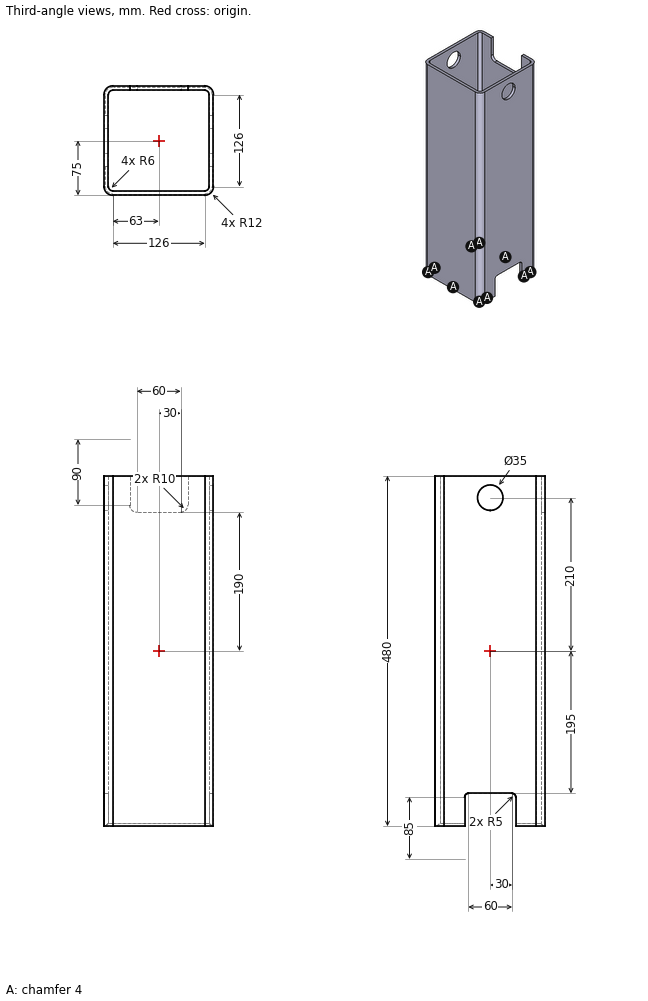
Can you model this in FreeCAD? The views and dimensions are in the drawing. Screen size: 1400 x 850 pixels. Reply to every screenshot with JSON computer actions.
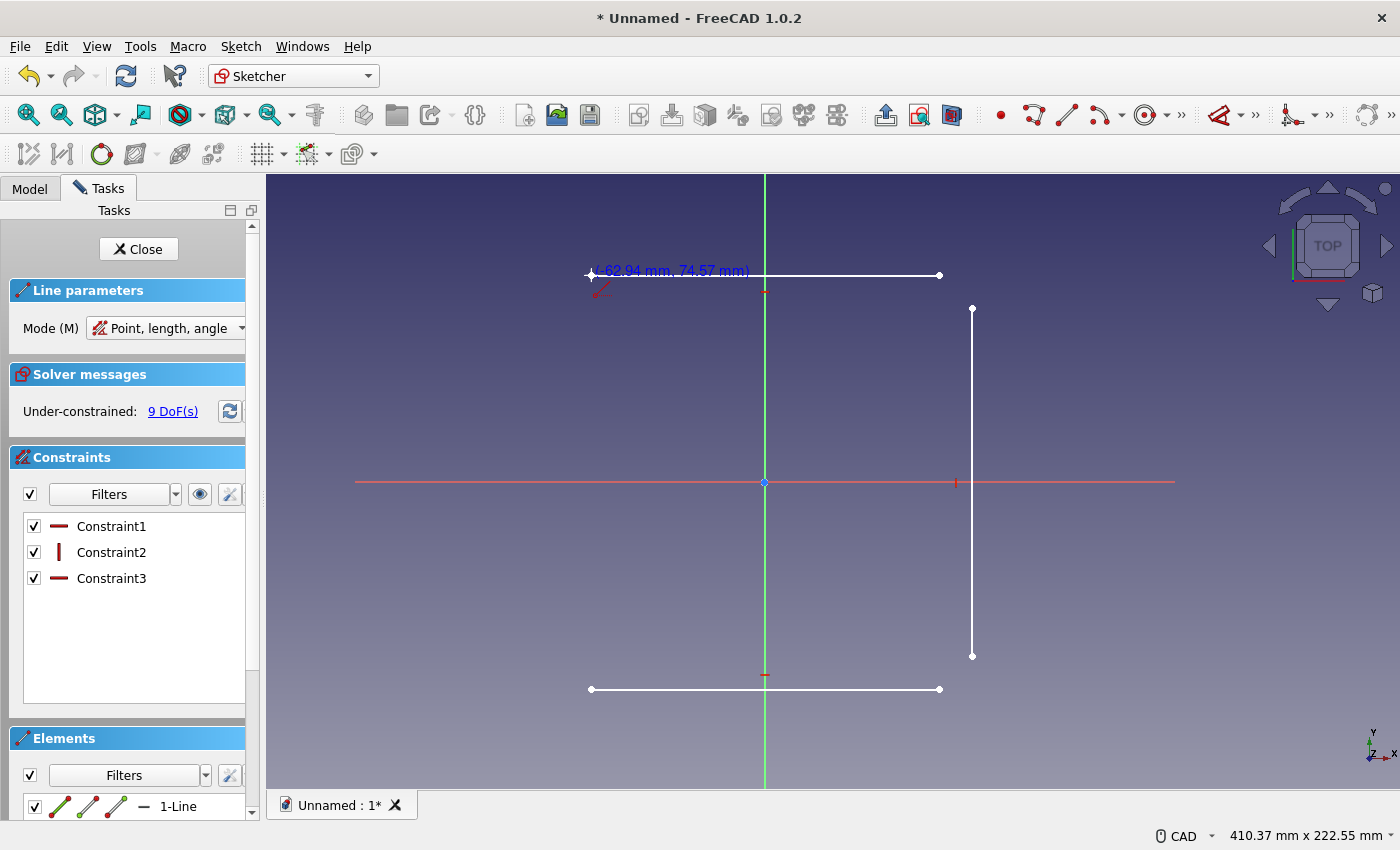
{"action": "left_click", "coordinate": [558, 308]}
{"action": "left_click", "coordinate": [558, 656]}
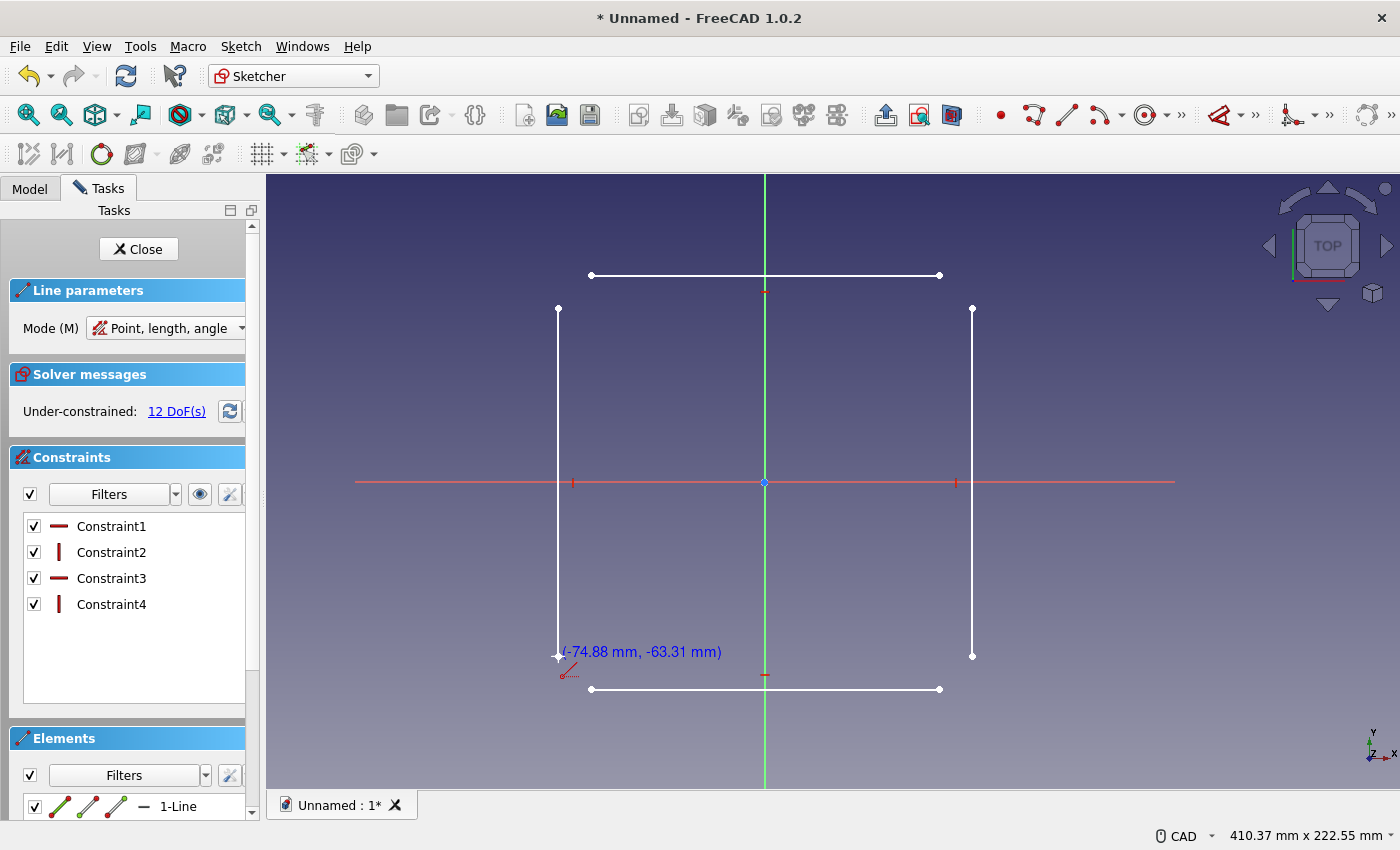
{"action": "key", "text": "g 3 a"}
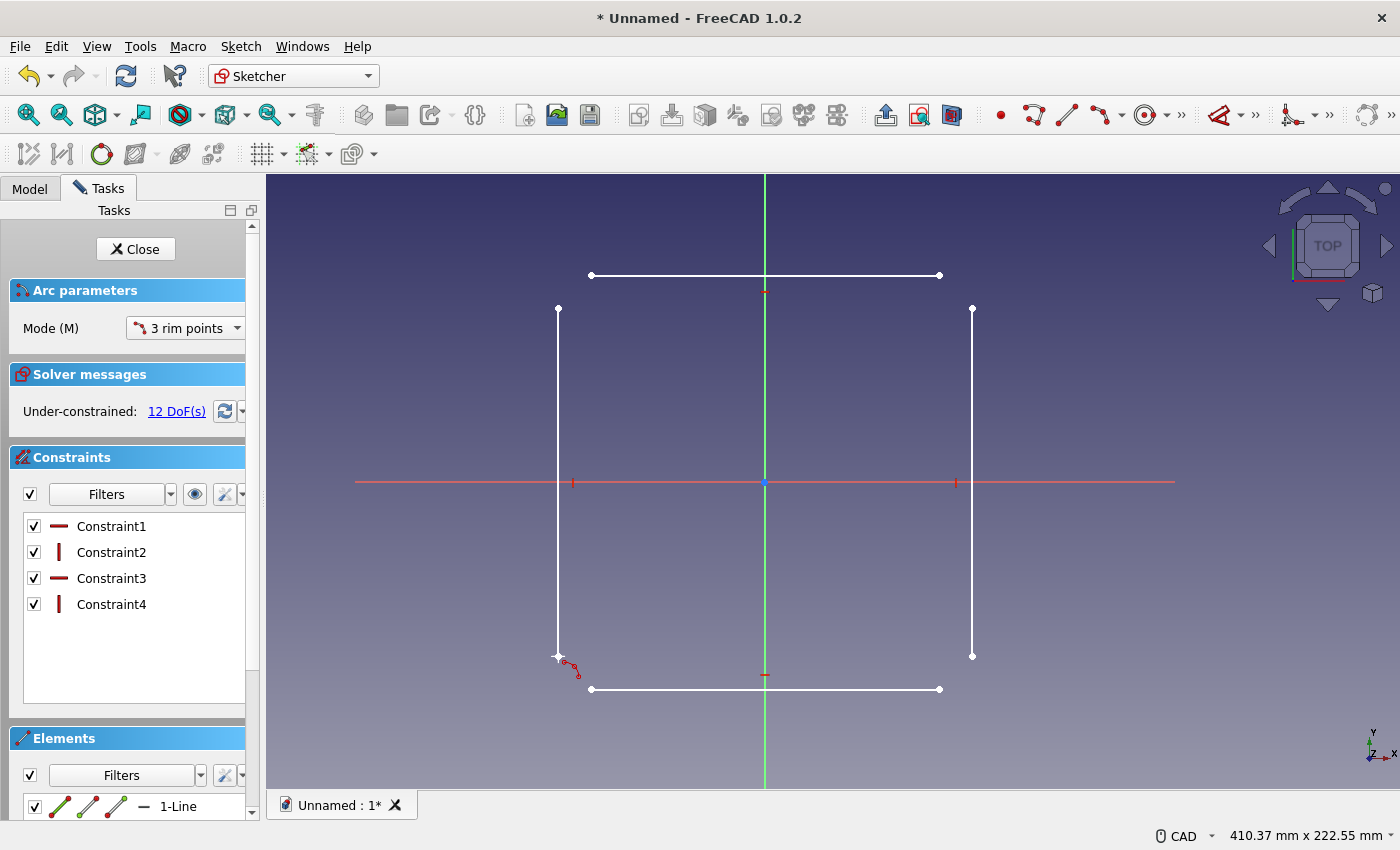
{"action": "left_click", "coordinate": [939, 690]}
{"action": "left_click", "coordinate": [972, 657]}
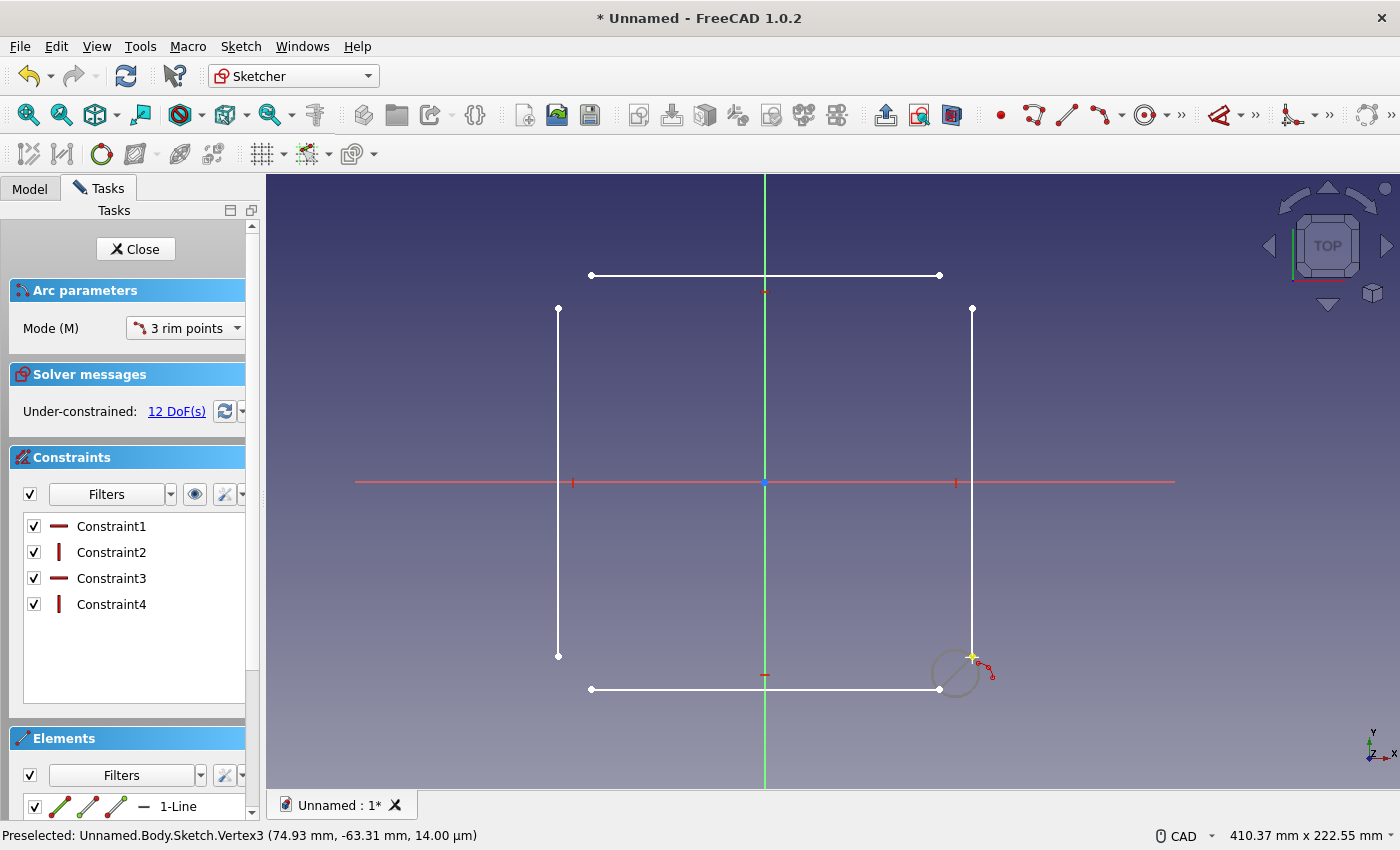
{"action": "scroll", "coordinate": [962, 680], "scroll_direction": "up", "scroll_amount": 3}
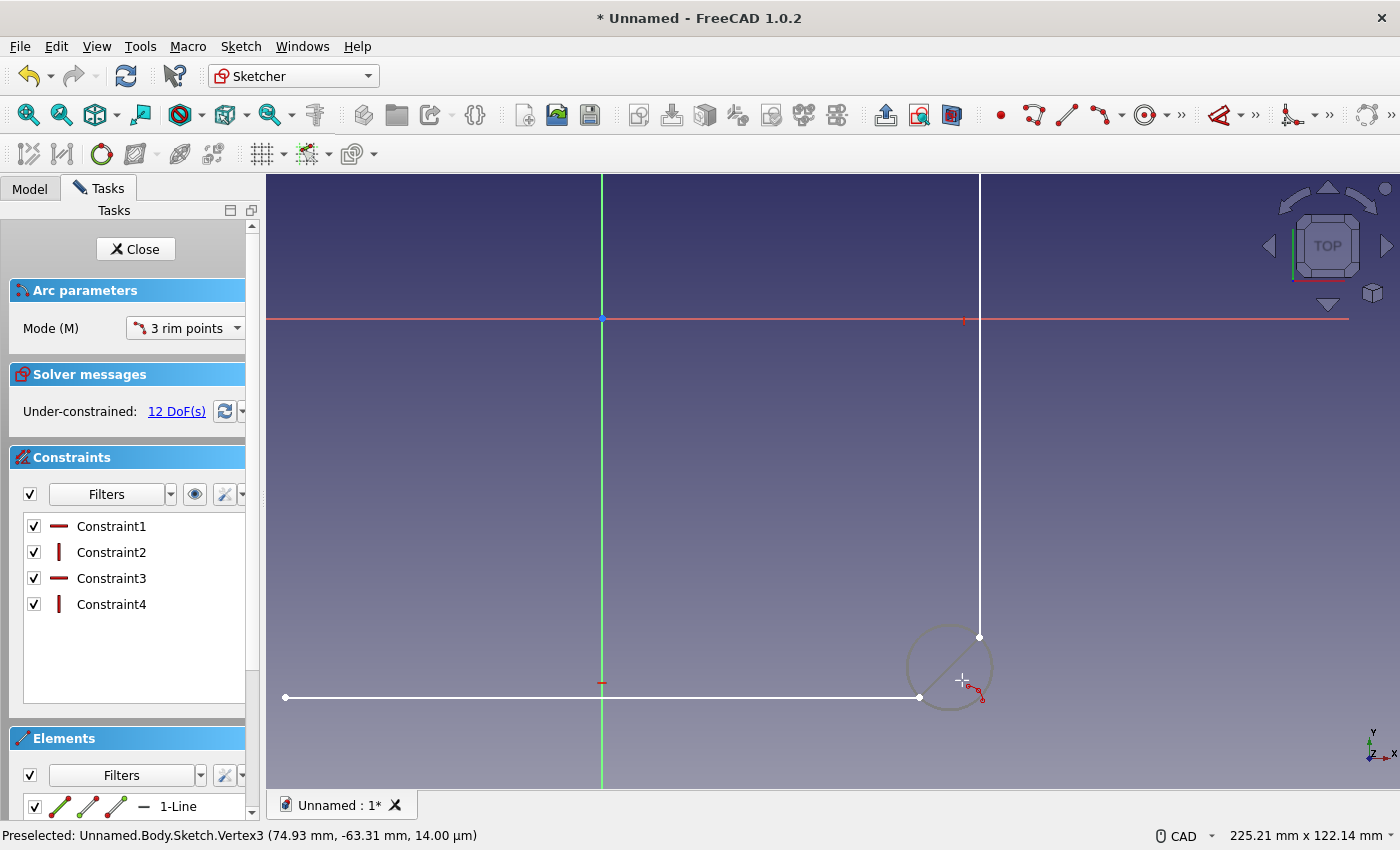
{"action": "left_click", "coordinate": [962, 679]}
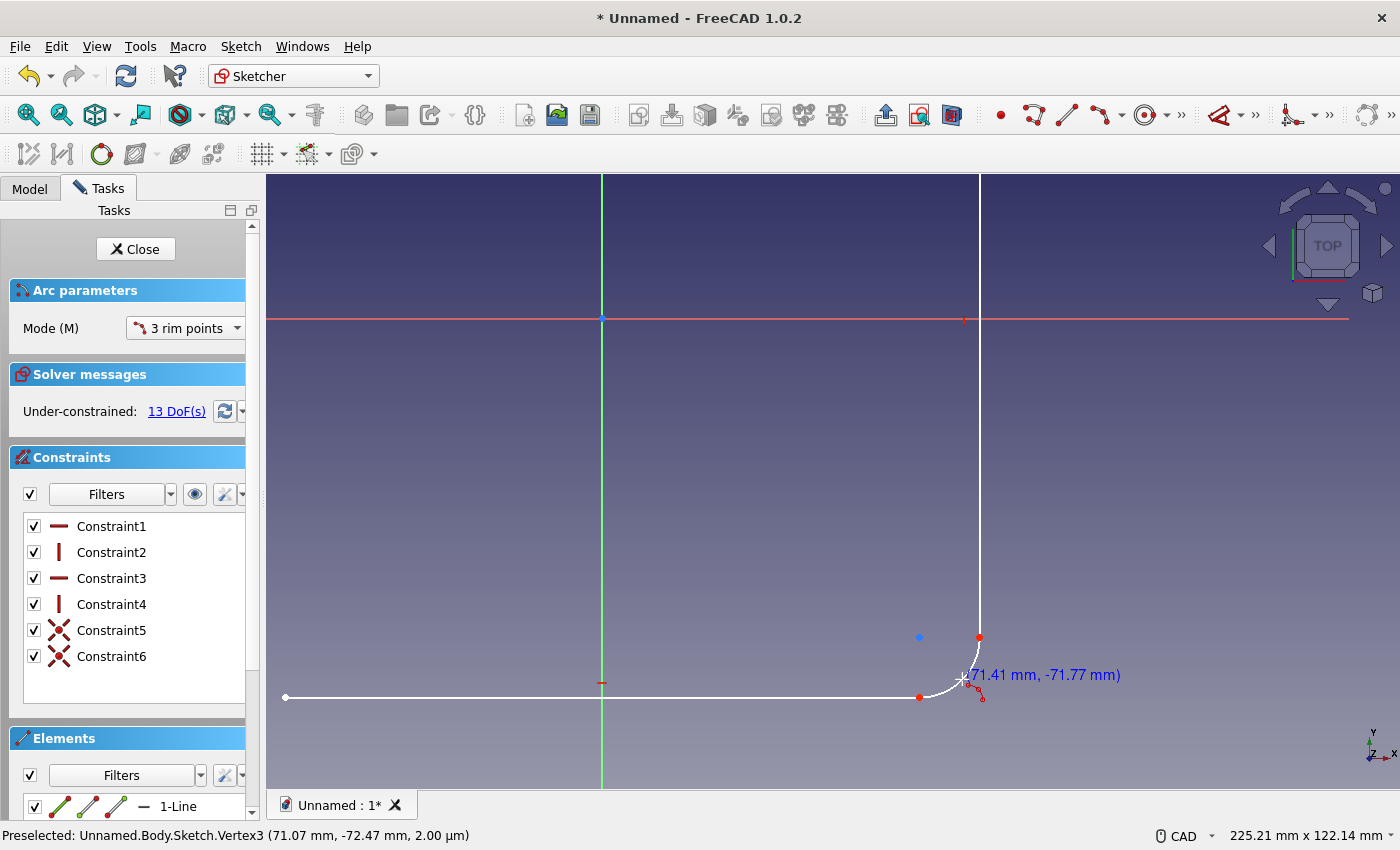
{"action": "scroll", "coordinate": [962, 680], "scroll_direction": "down", "scroll_amount": 3}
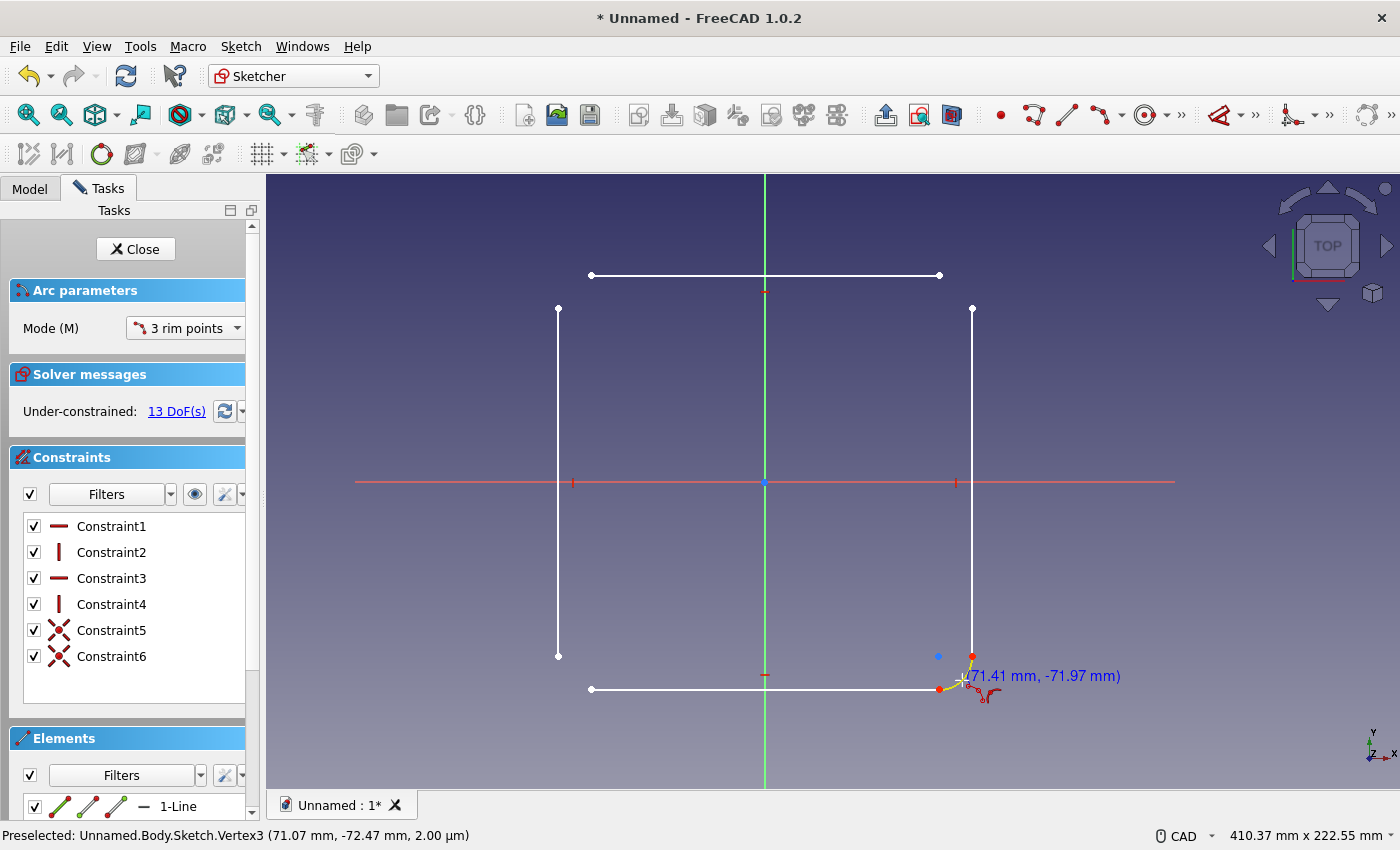
{"action": "left_click", "coordinate": [972, 309]}
{"action": "left_click", "coordinate": [939, 276]}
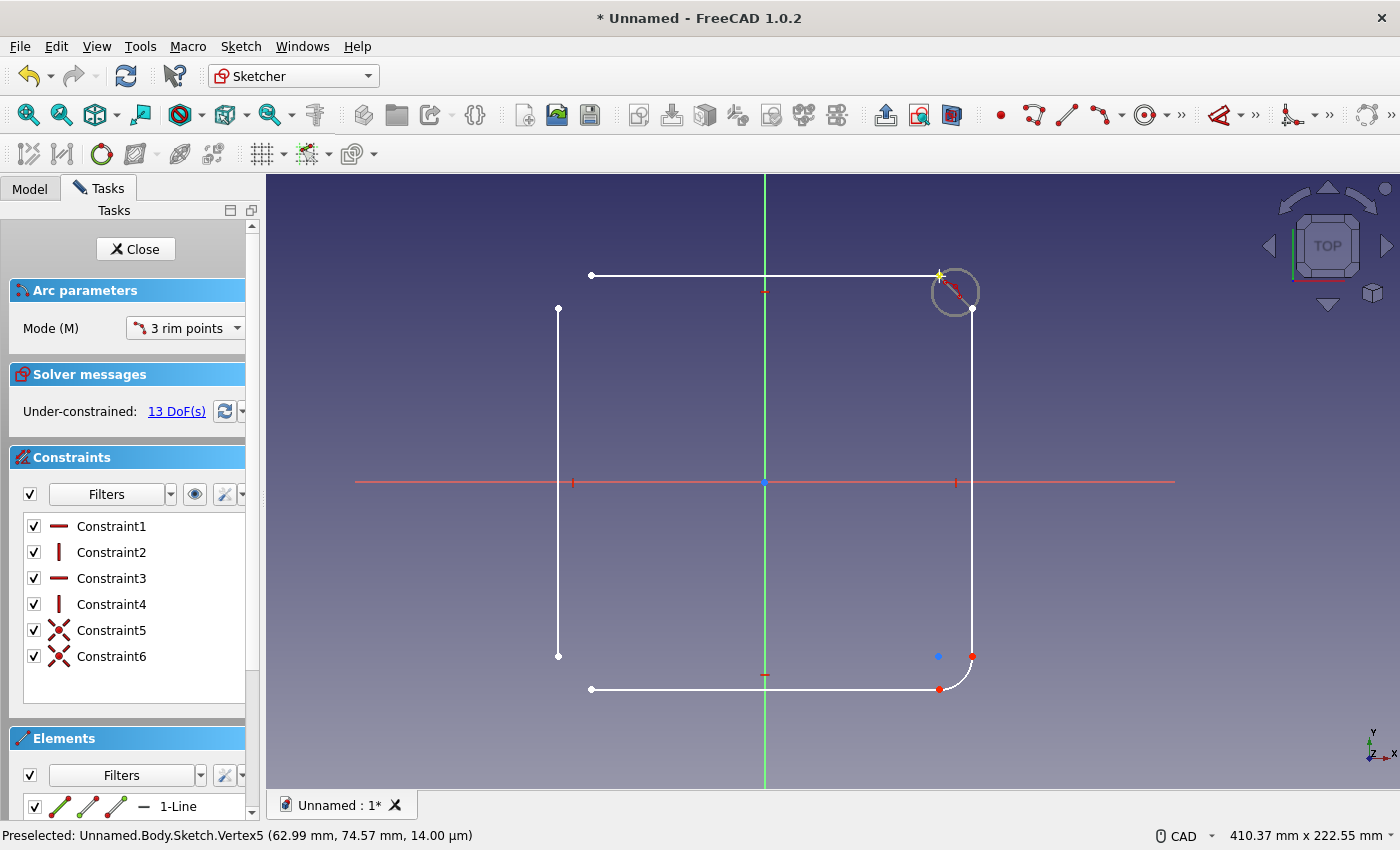
{"action": "scroll", "coordinate": [962, 285], "scroll_direction": "up", "scroll_amount": 3}